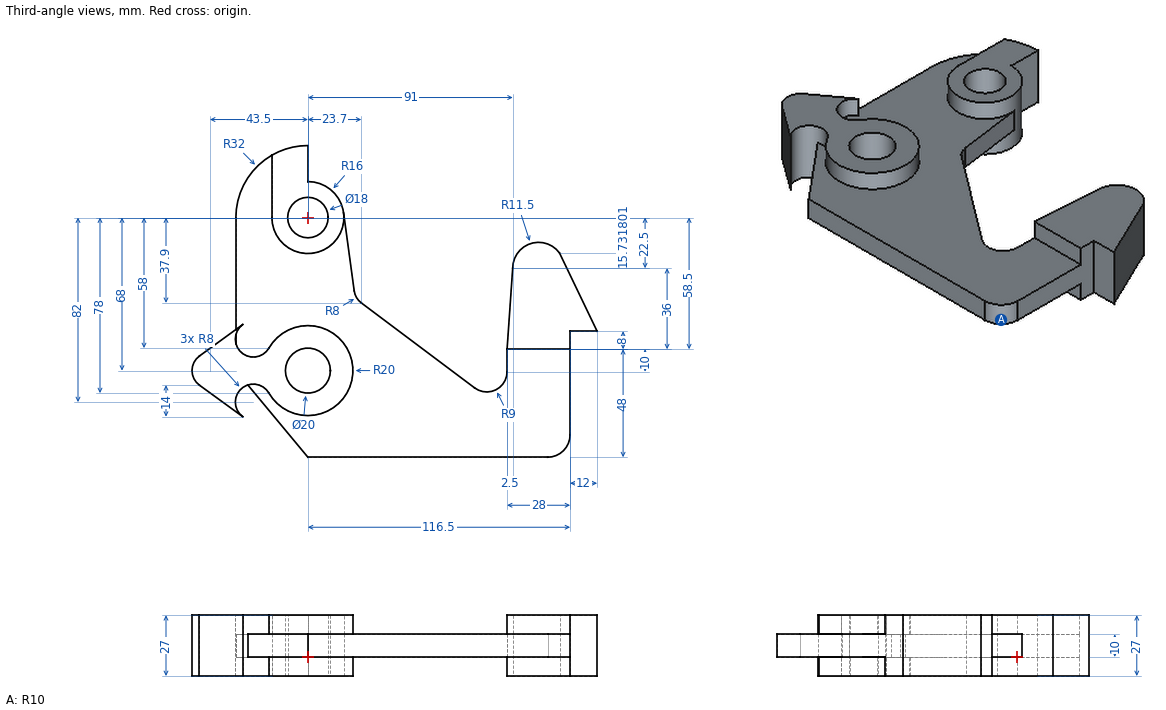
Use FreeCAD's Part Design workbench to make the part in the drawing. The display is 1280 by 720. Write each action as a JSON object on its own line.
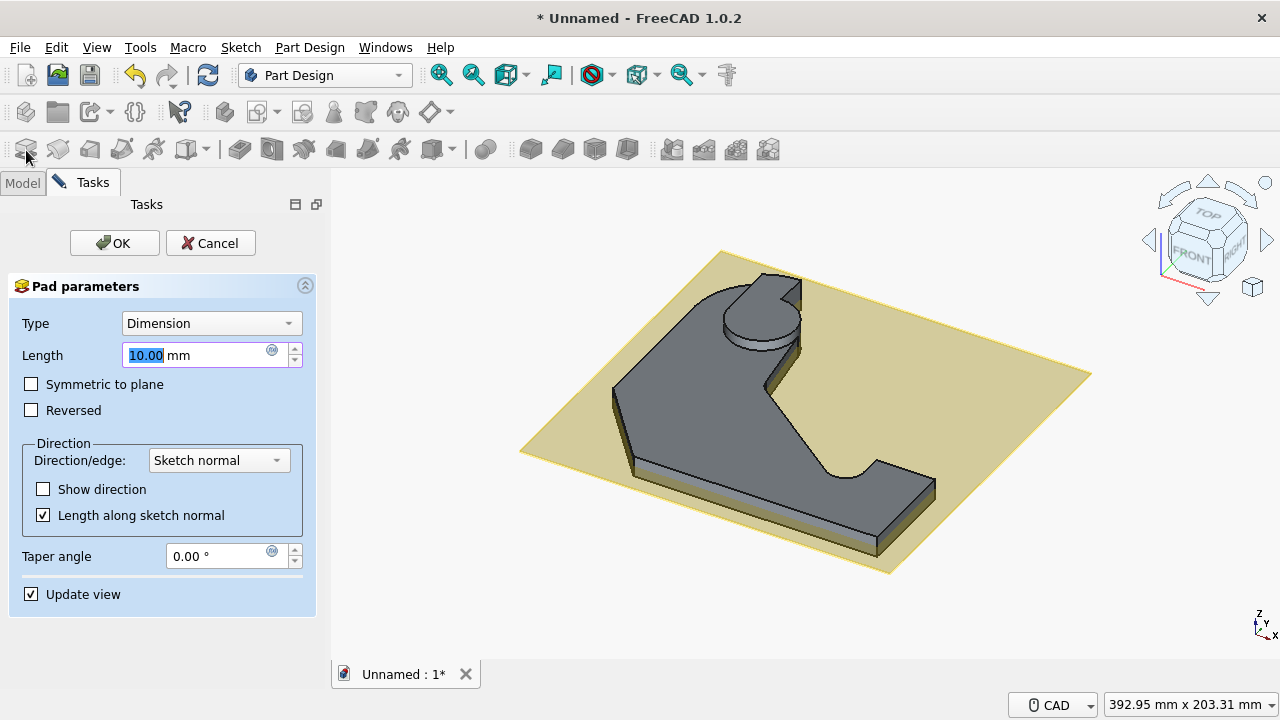
{"action": "type", "text": "27"}
{"action": "key", "text": "Tab"}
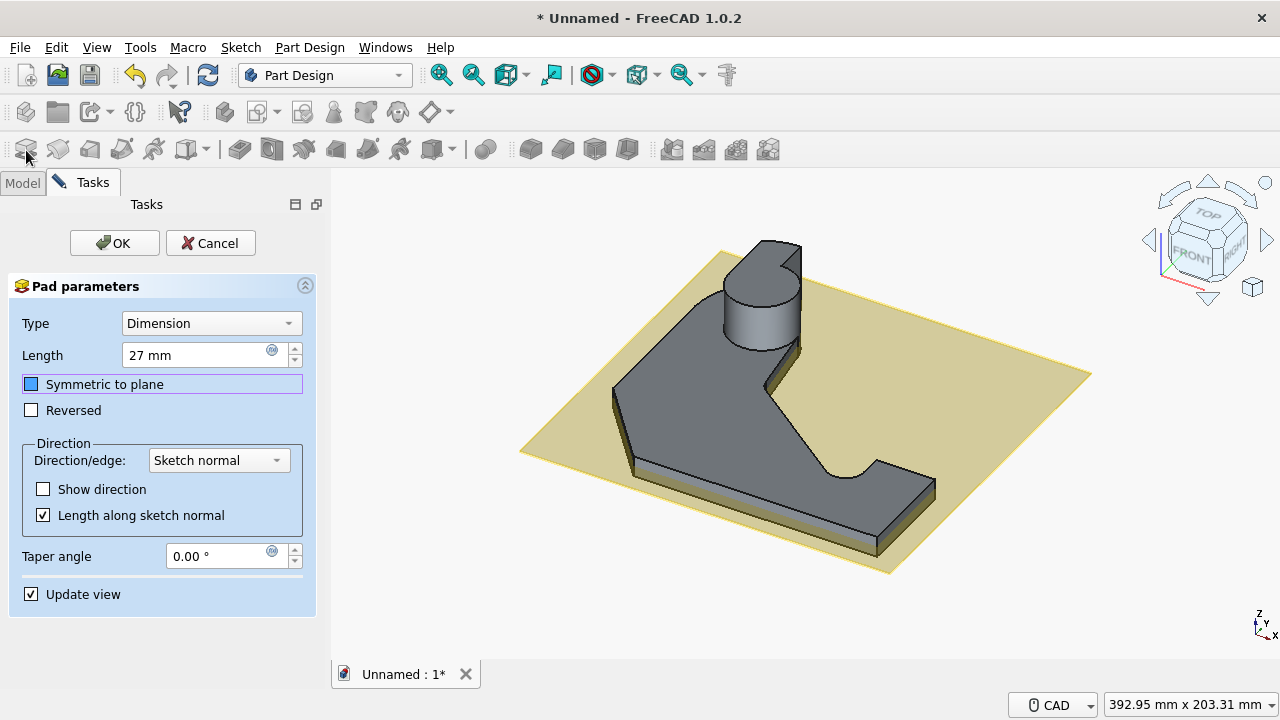
{"action": "left_click", "coordinate": [30, 384]}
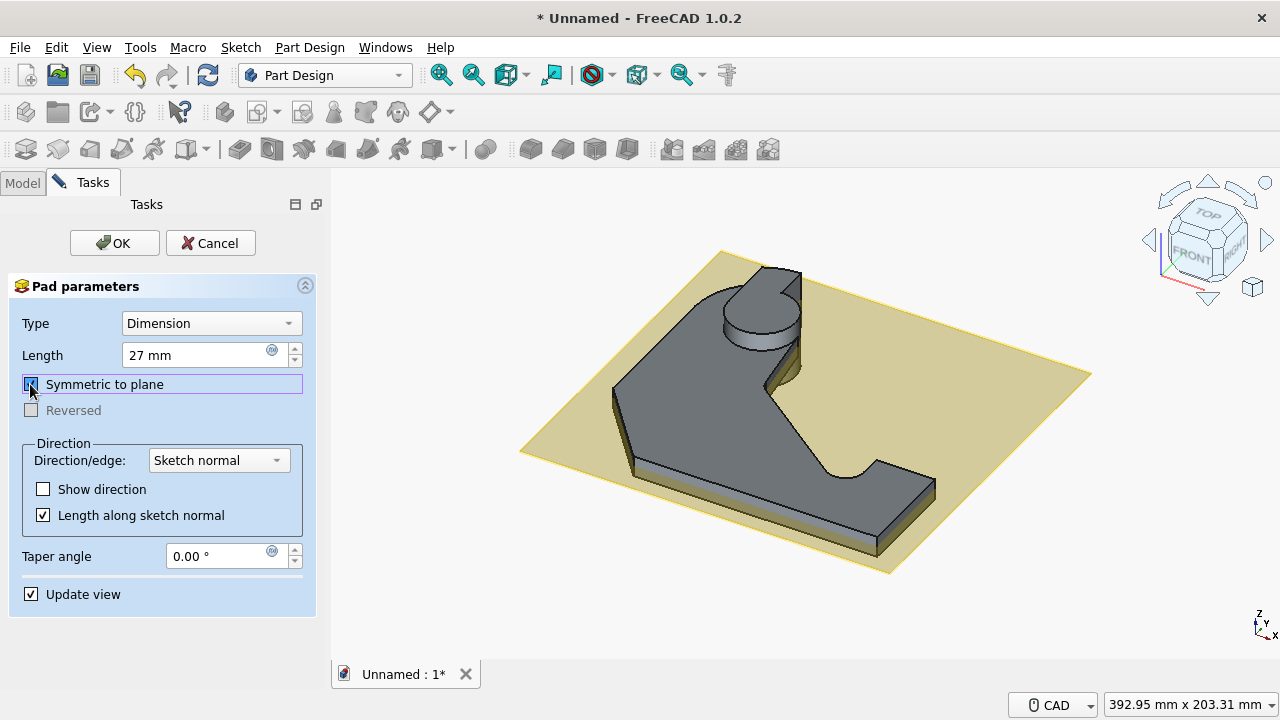
{"action": "left_click", "coordinate": [115, 243]}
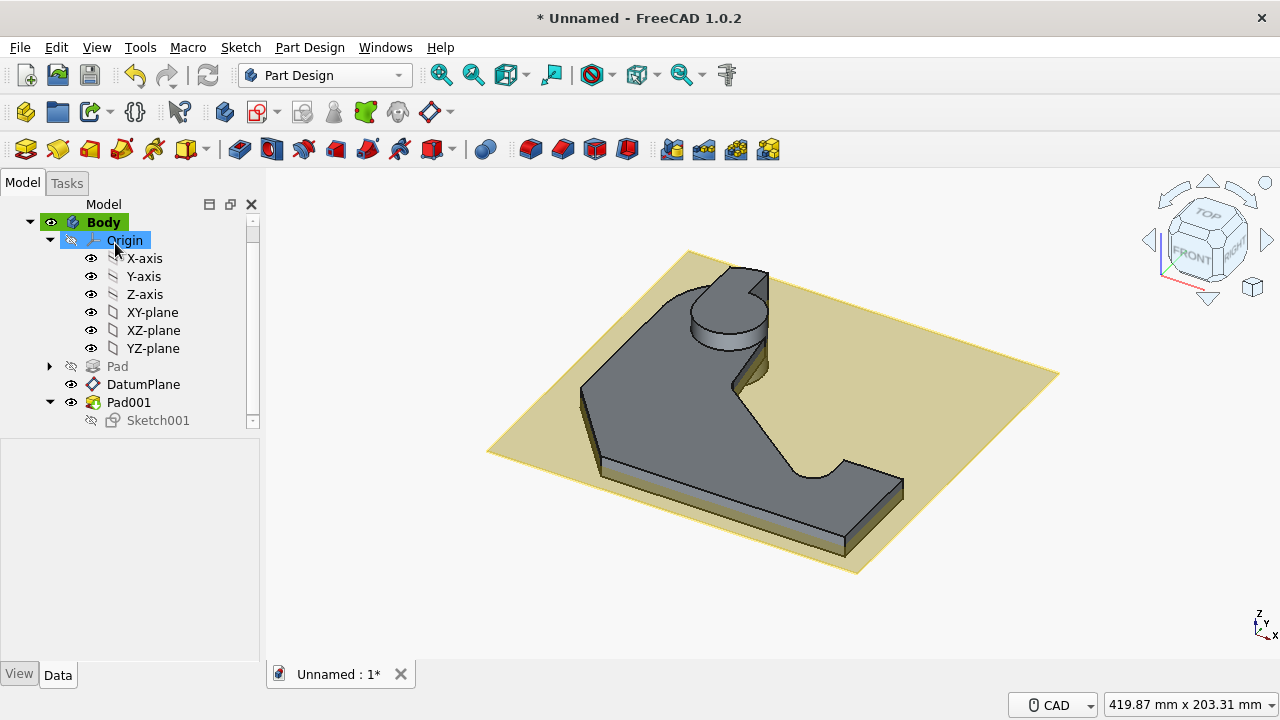
{"action": "left_click", "coordinate": [116, 384]}
{"action": "key", "text": "space"}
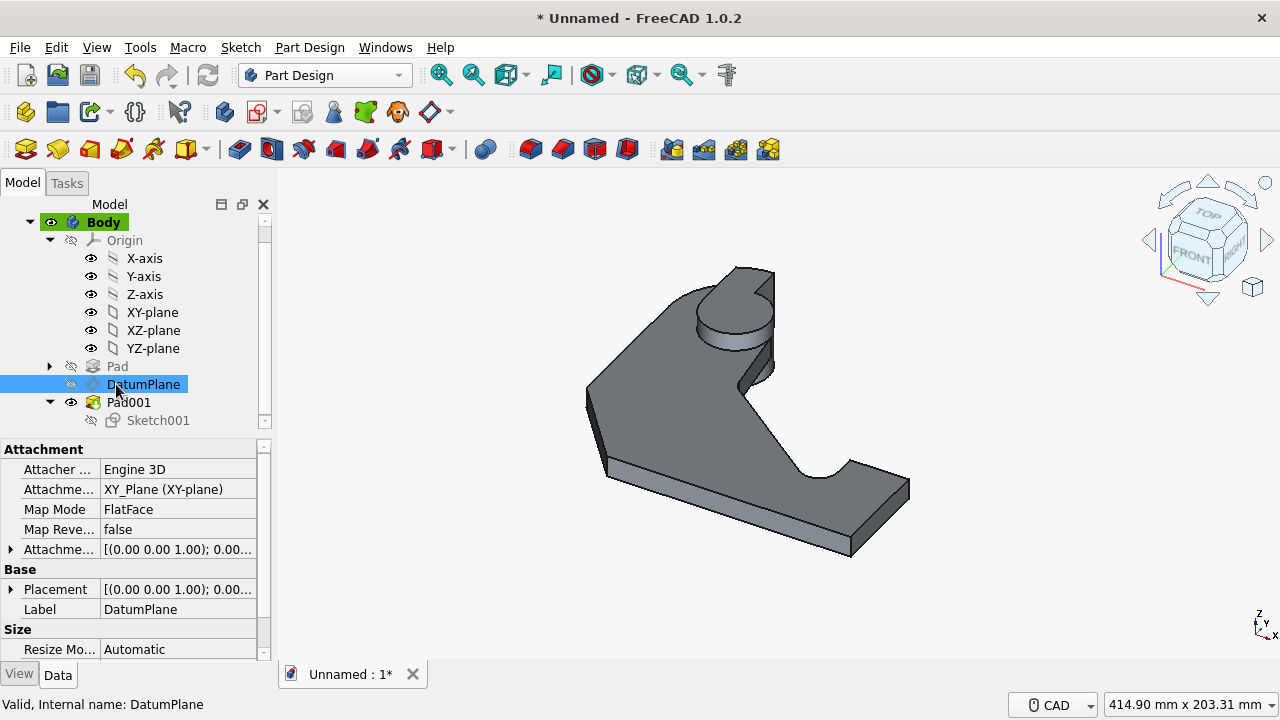
{"action": "left_click", "coordinate": [737, 309]}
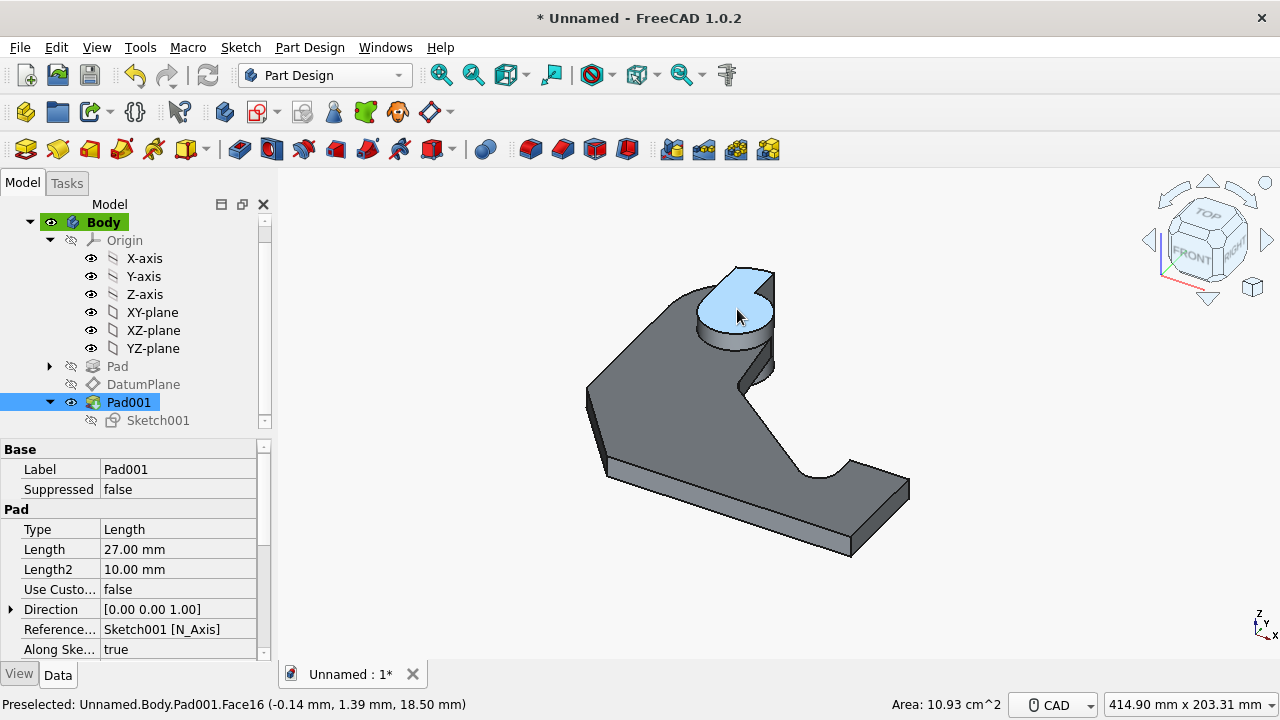
{"action": "left_click", "coordinate": [258, 112]}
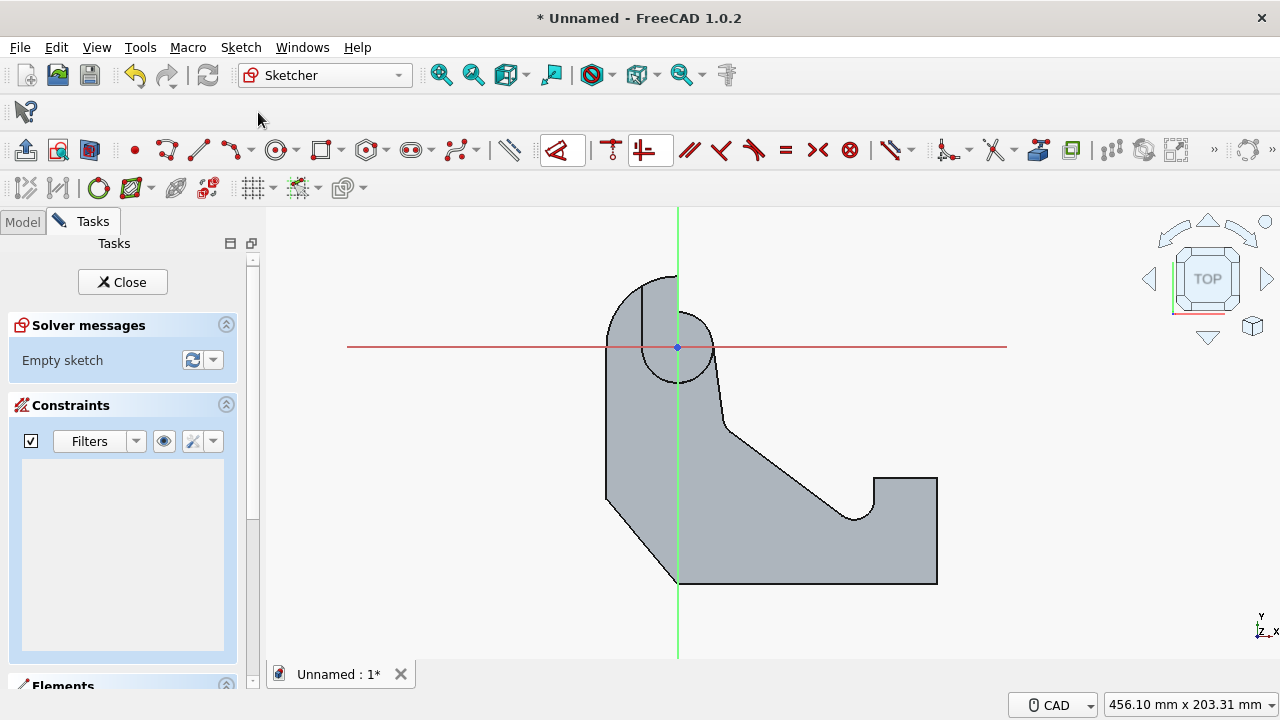
{"action": "scroll", "coordinate": [673, 334], "scroll_direction": "up", "scroll_amount": 10}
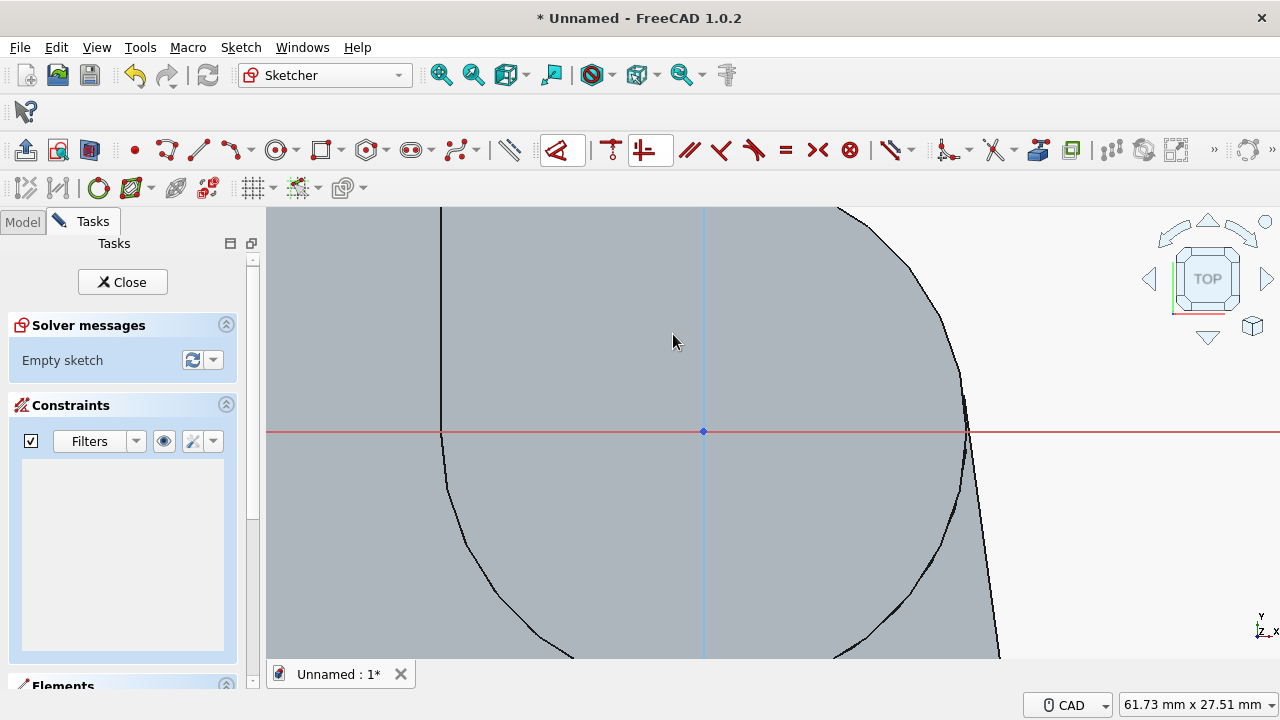
{"action": "left_click", "coordinate": [276, 150]}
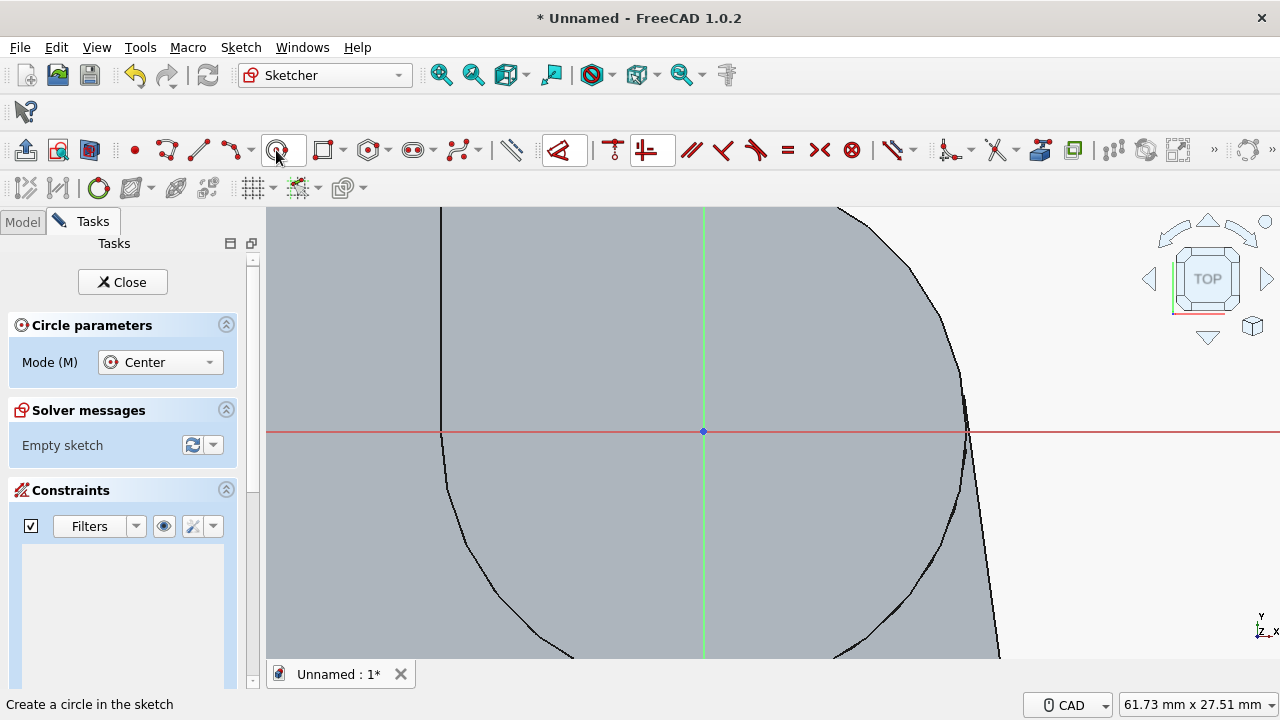
{"action": "left_click", "coordinate": [704, 432]}
{"action": "mouse_move", "coordinate": [808, 327]}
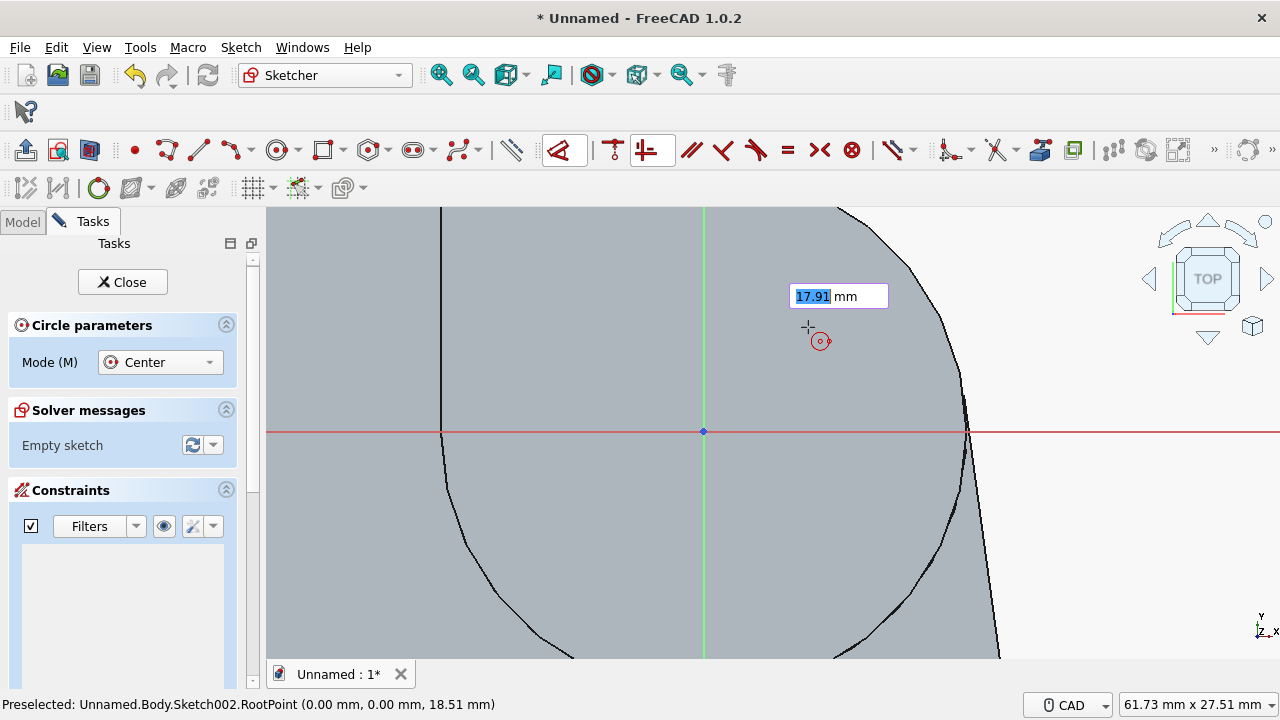
{"action": "type", "text": "18"}
{"action": "key", "text": "Return"}
{"action": "key", "text": "Escape"}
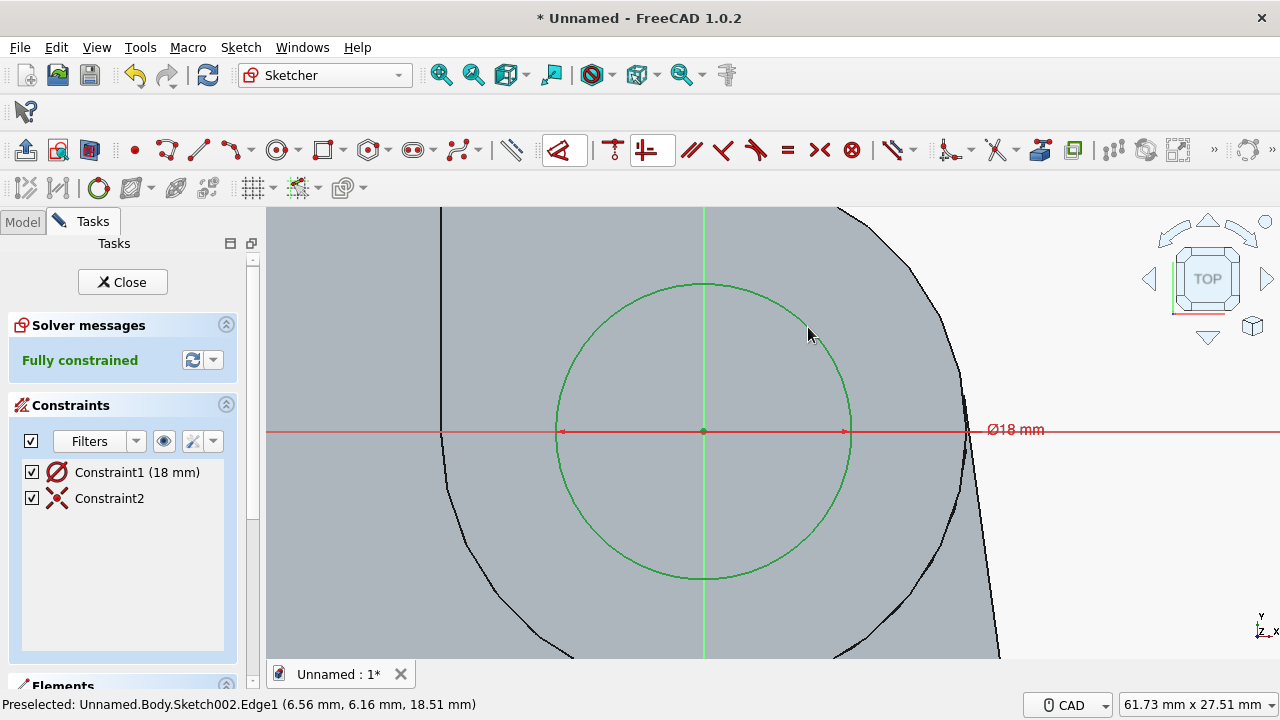
{"action": "left_click", "coordinate": [123, 282]}